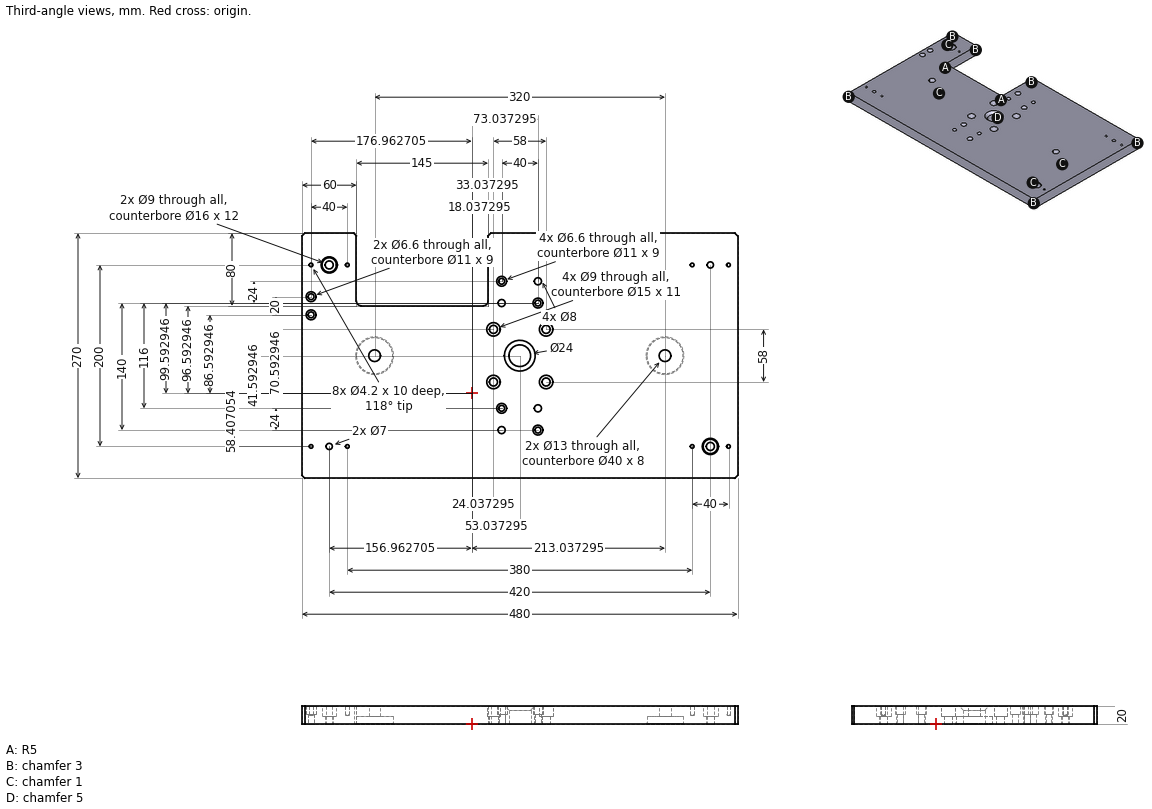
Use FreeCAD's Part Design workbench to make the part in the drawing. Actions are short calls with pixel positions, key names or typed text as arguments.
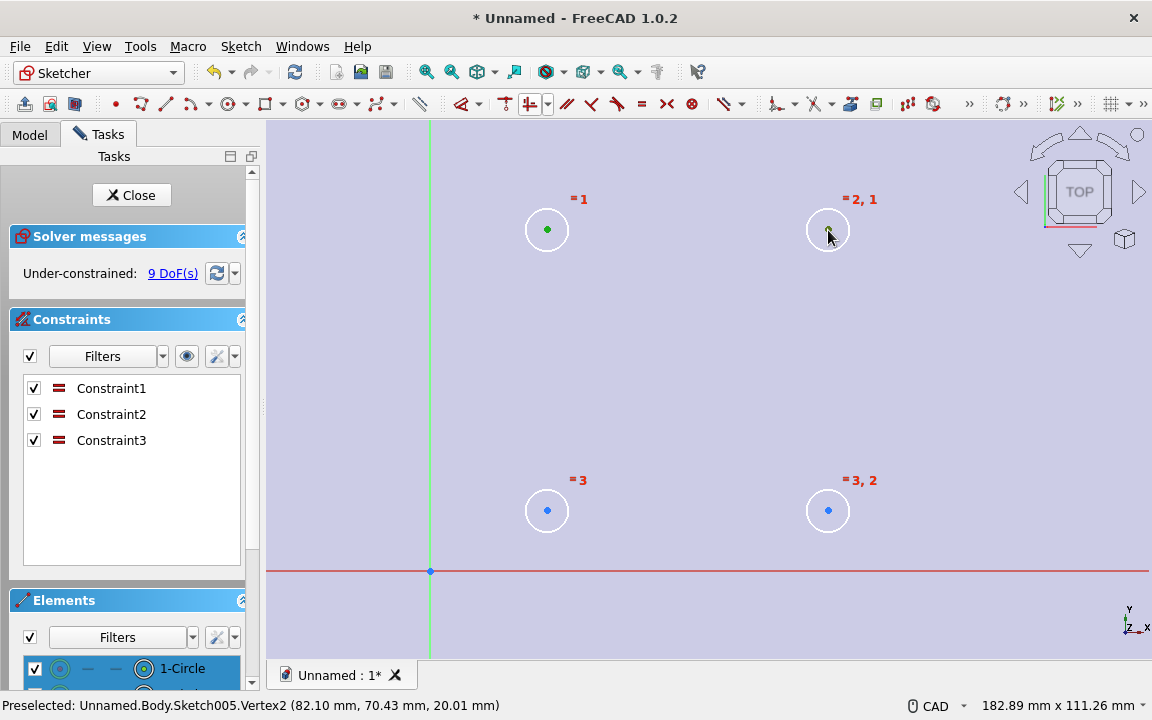
key(h)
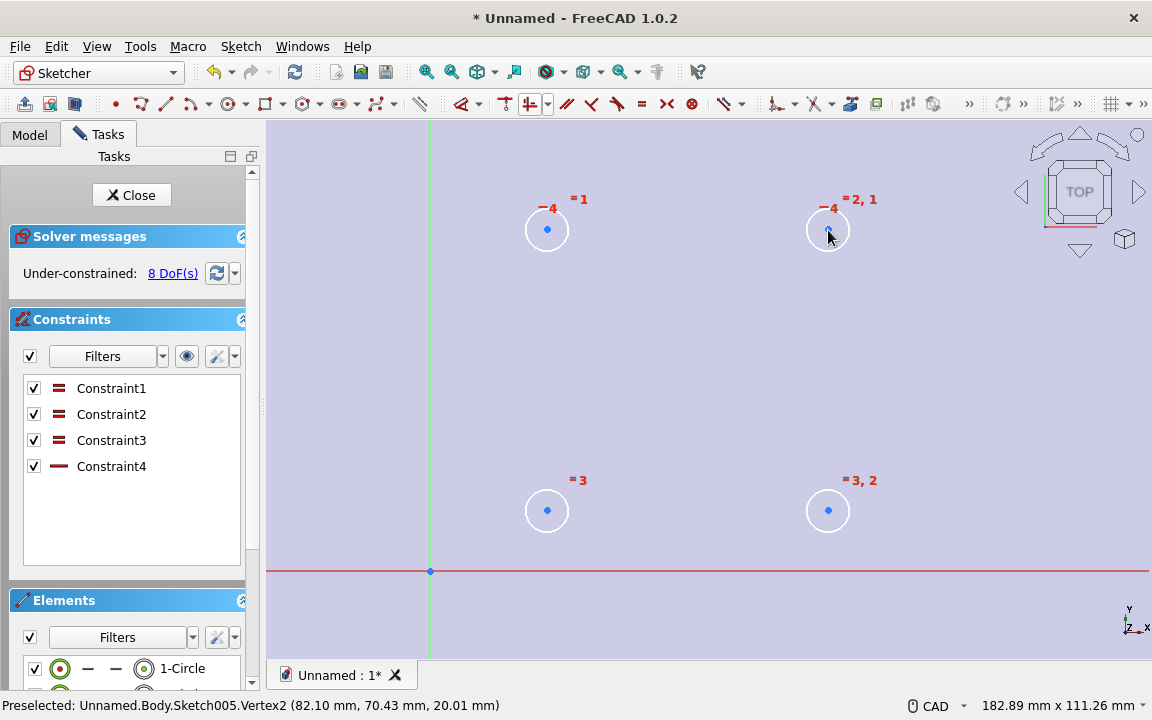
click(828, 230)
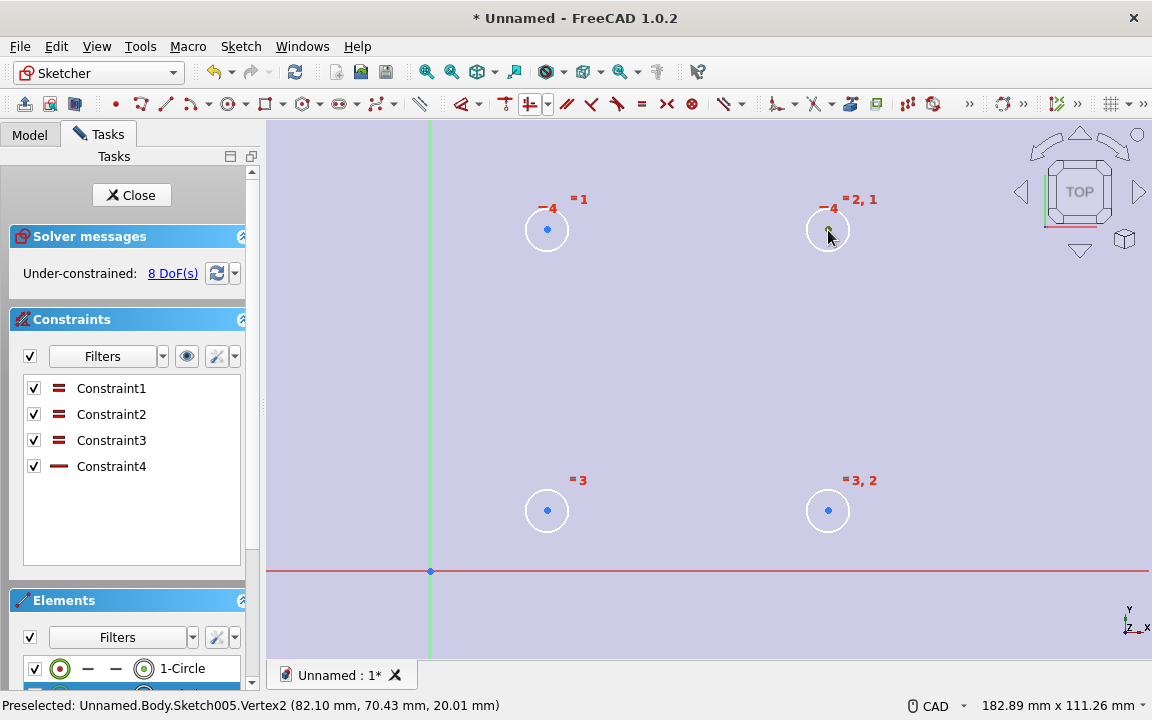
click(828, 511)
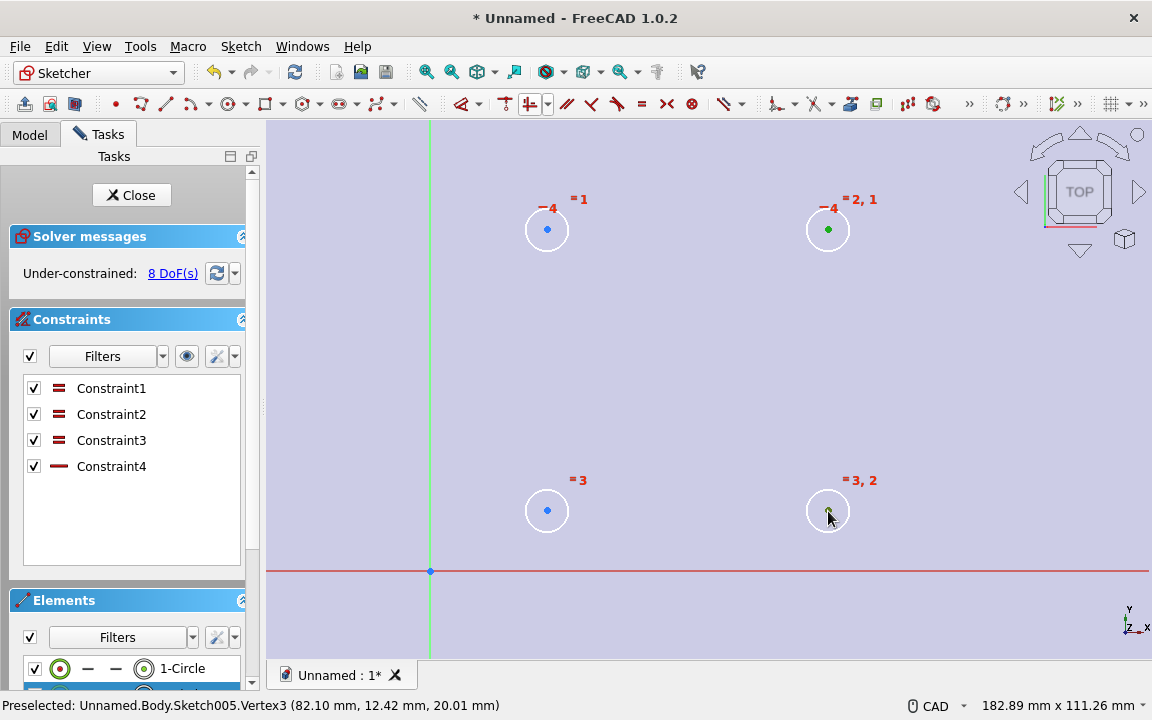
key(v)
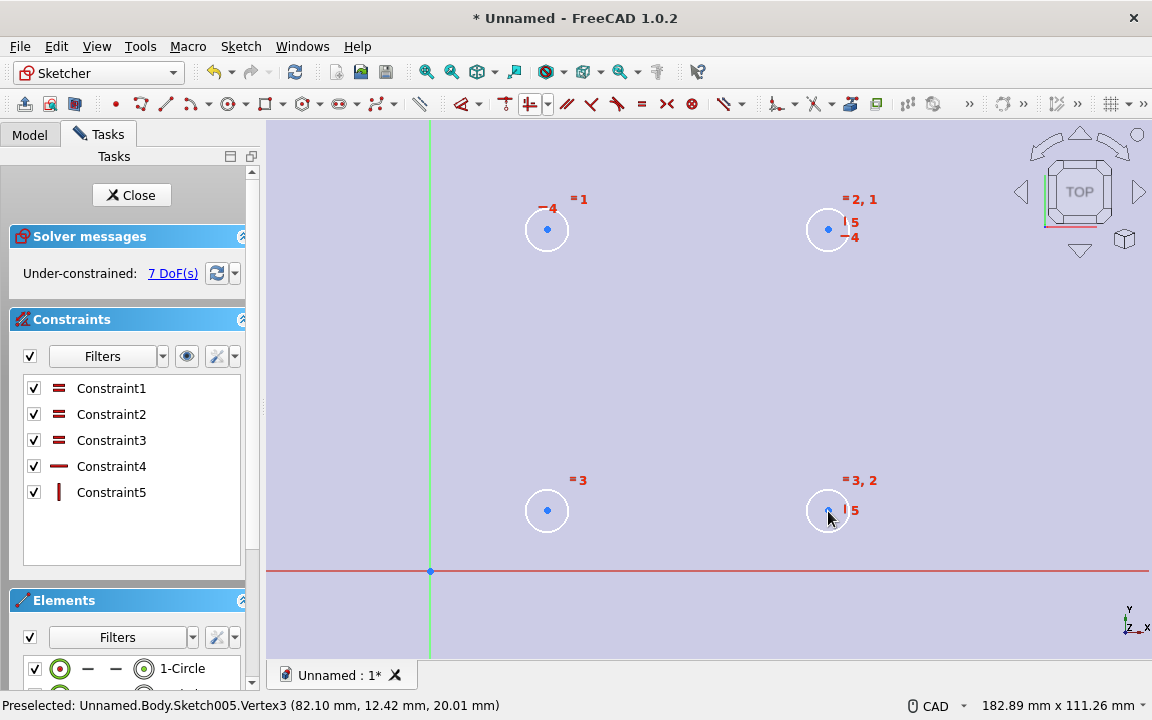
click(547, 230)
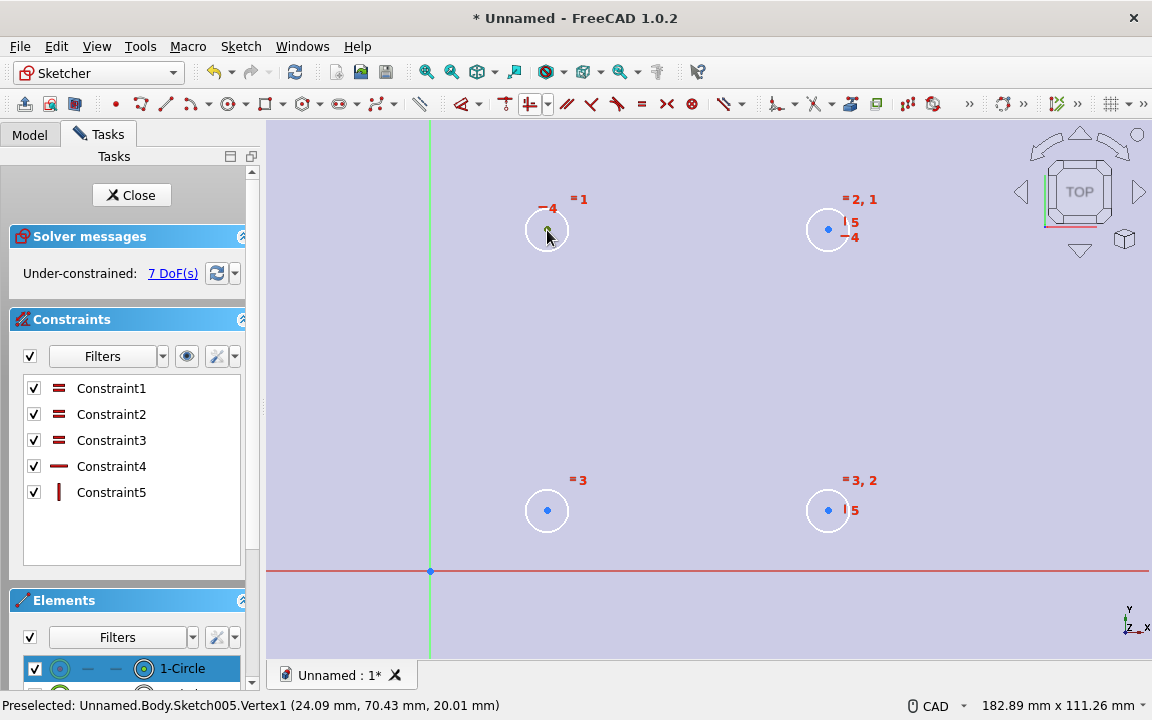
click(547, 511)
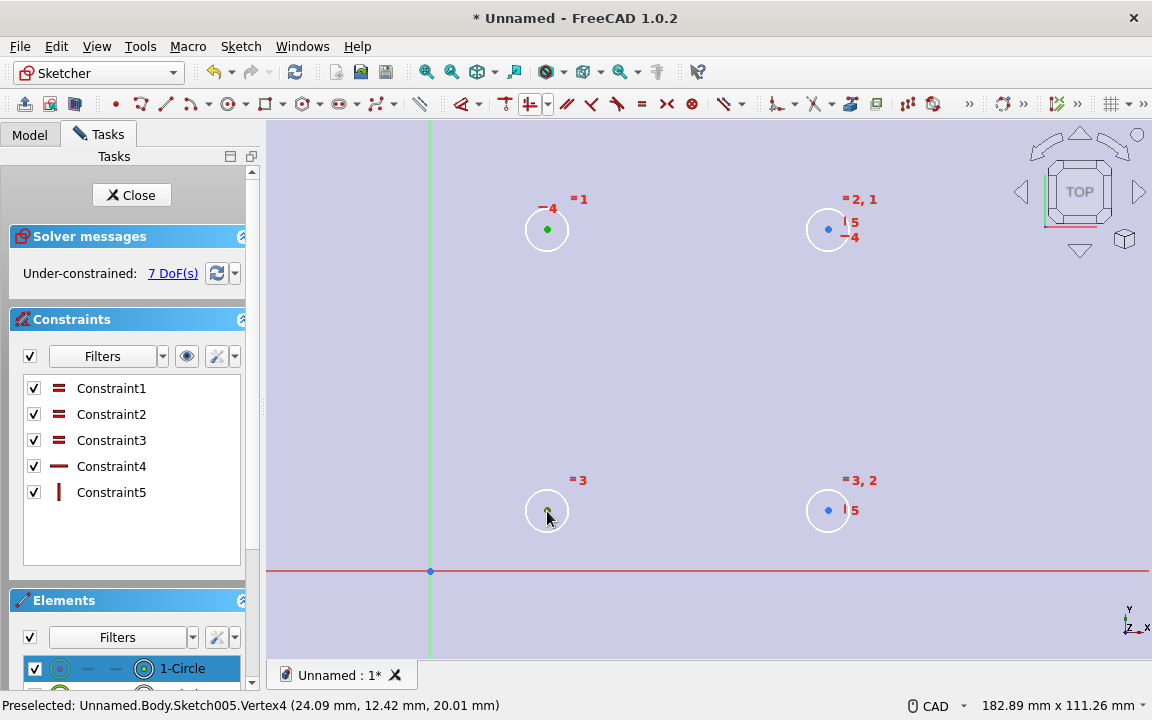
key(v)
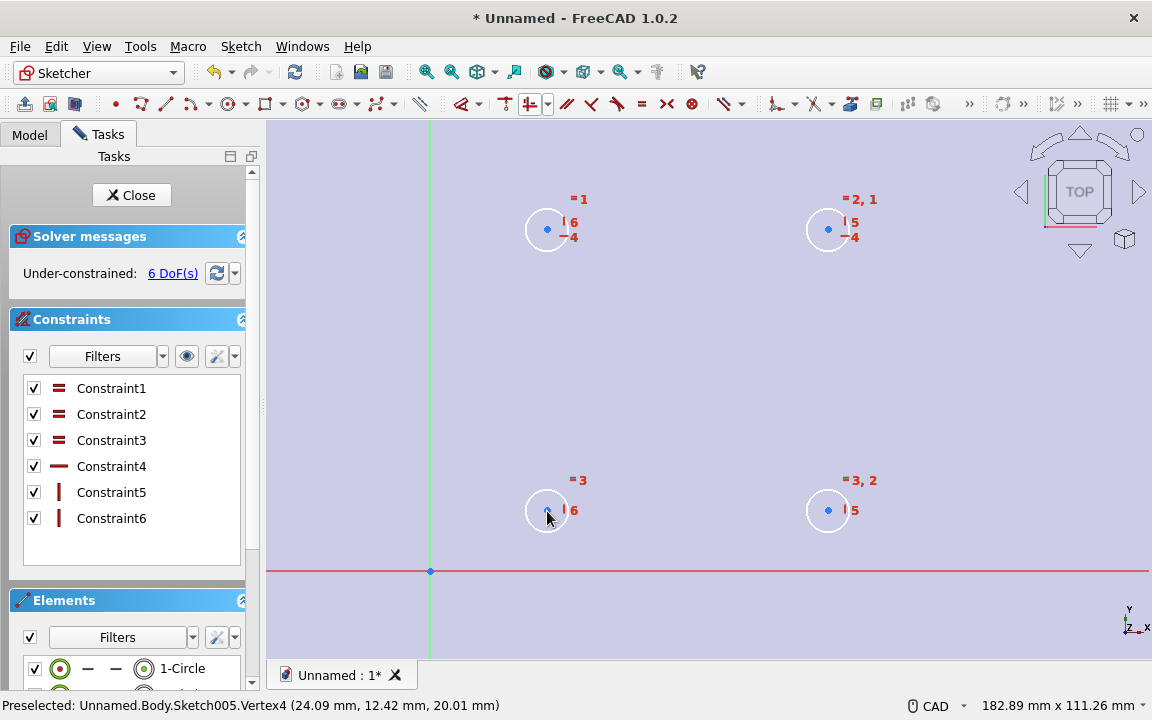
click(828, 511)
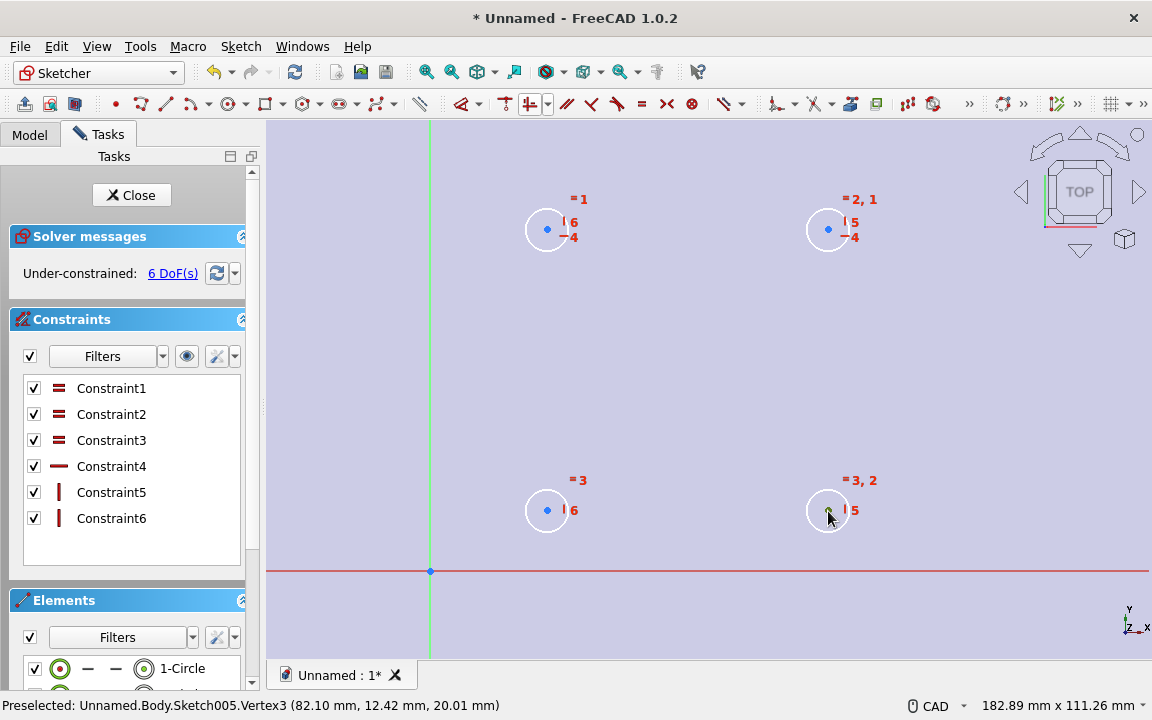
click(547, 511)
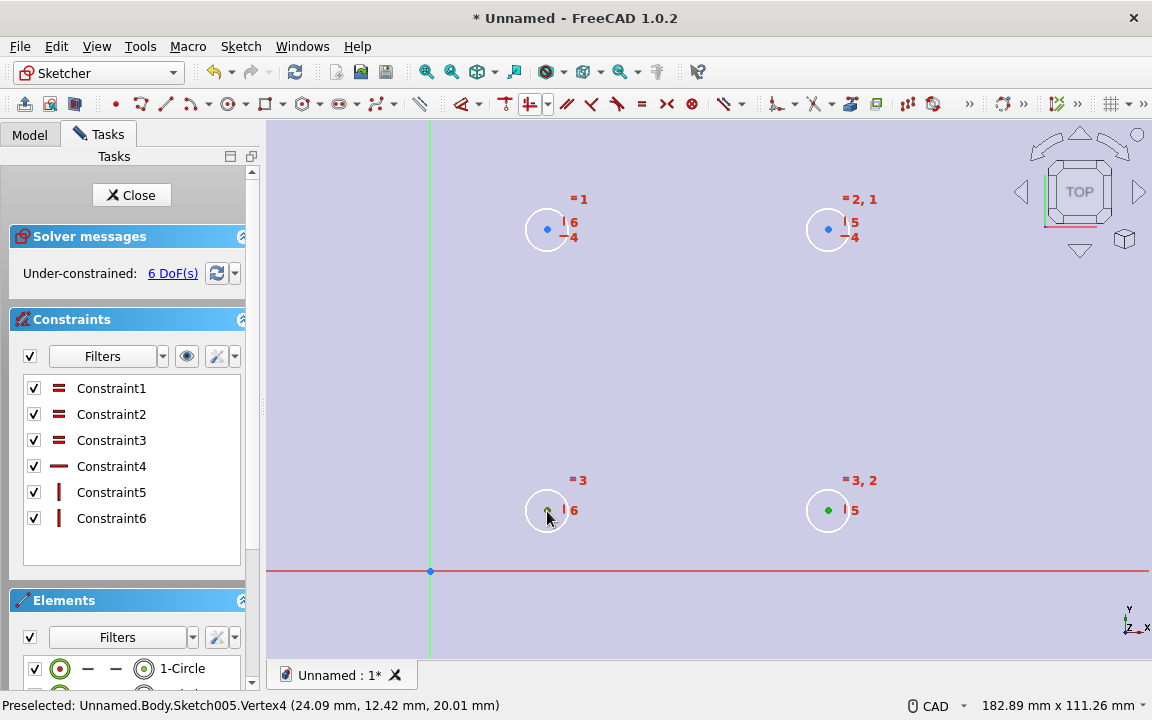
key(h)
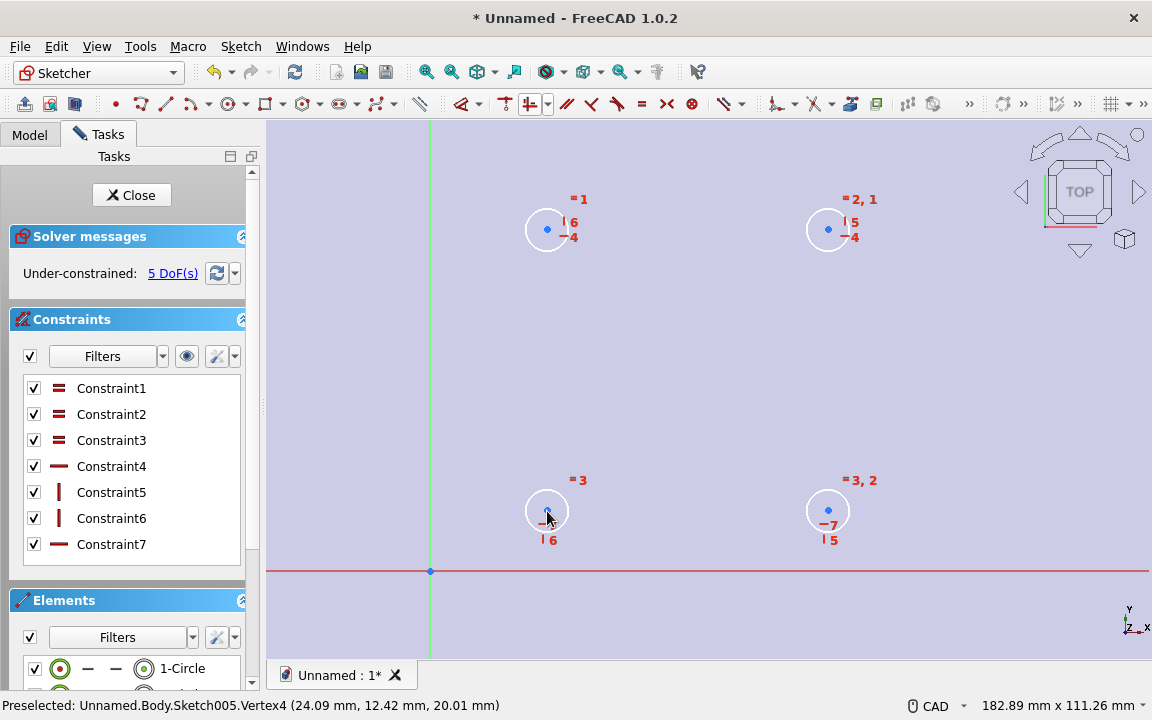
click(460, 104)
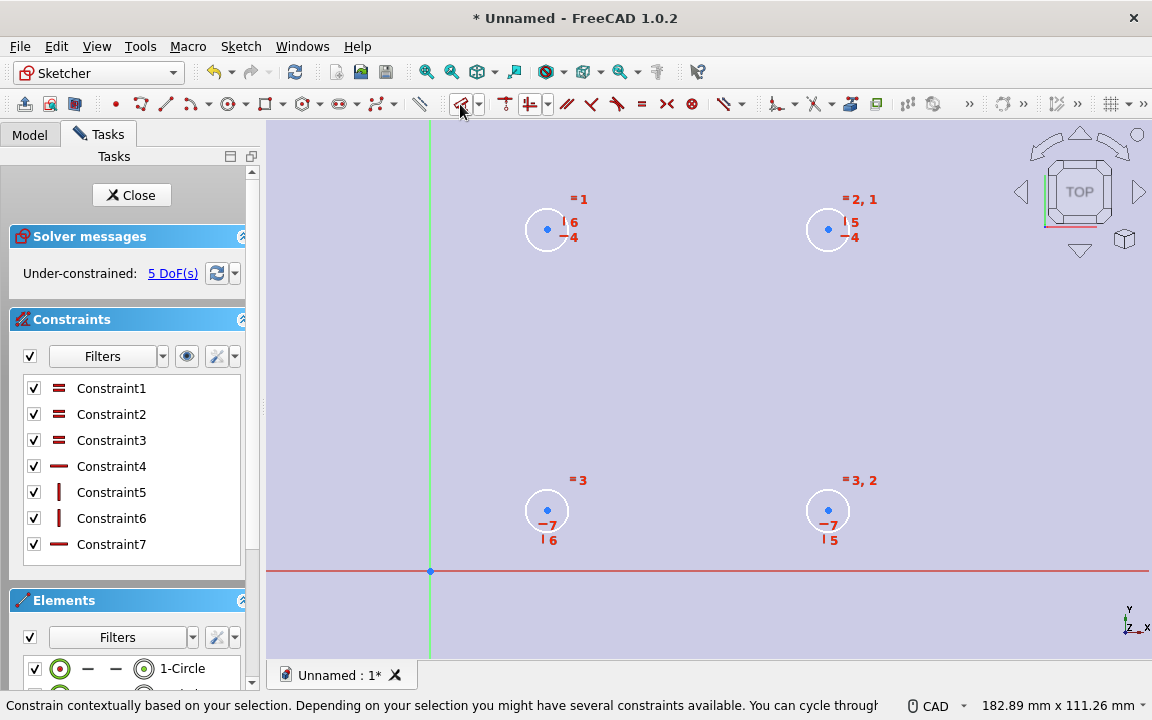
click(562, 215)
click(585, 192)